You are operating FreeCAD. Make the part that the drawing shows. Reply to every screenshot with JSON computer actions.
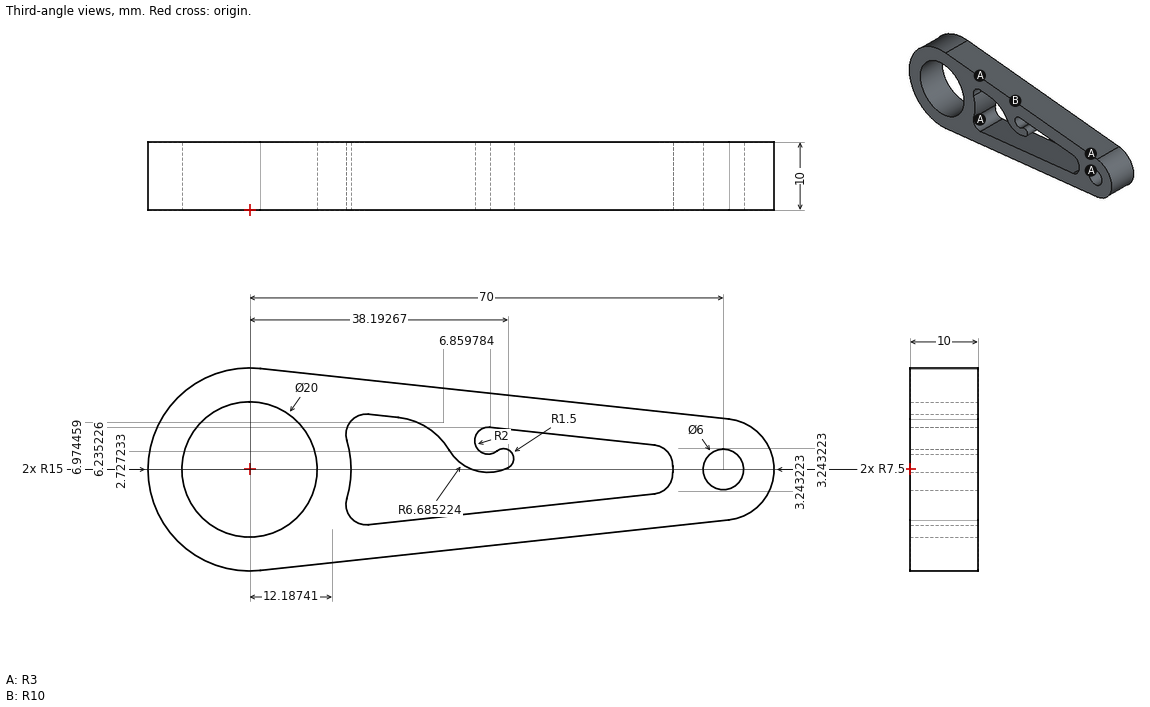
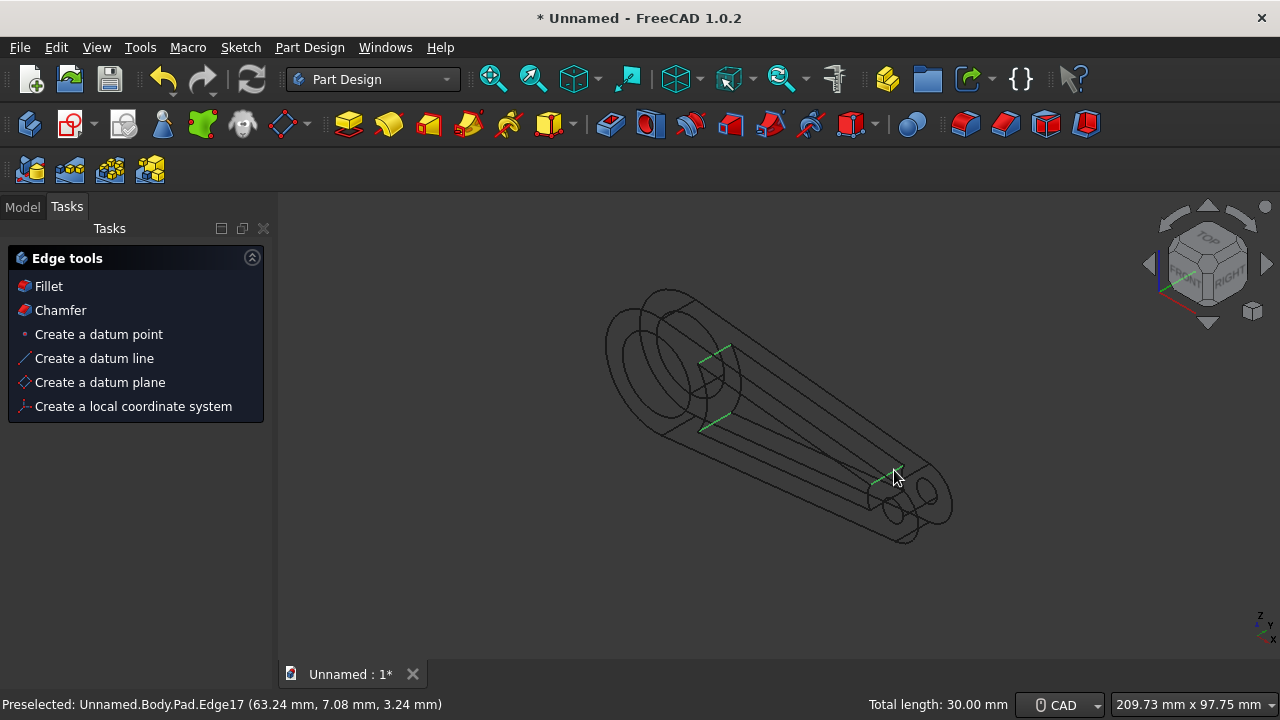
{"action": "scroll", "coordinate": [887, 500], "scroll_direction": "up", "scroll_amount": 6}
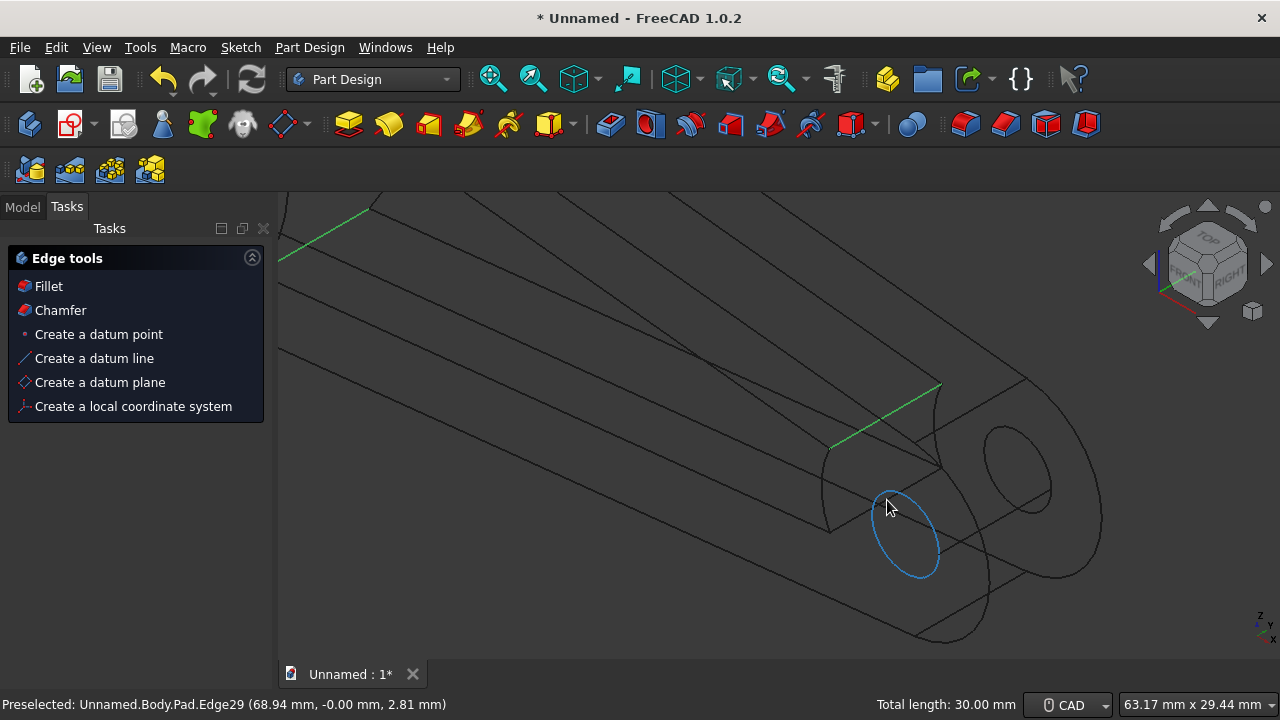
{"action": "left_click", "coordinate": [886, 499], "text": "ctrl"}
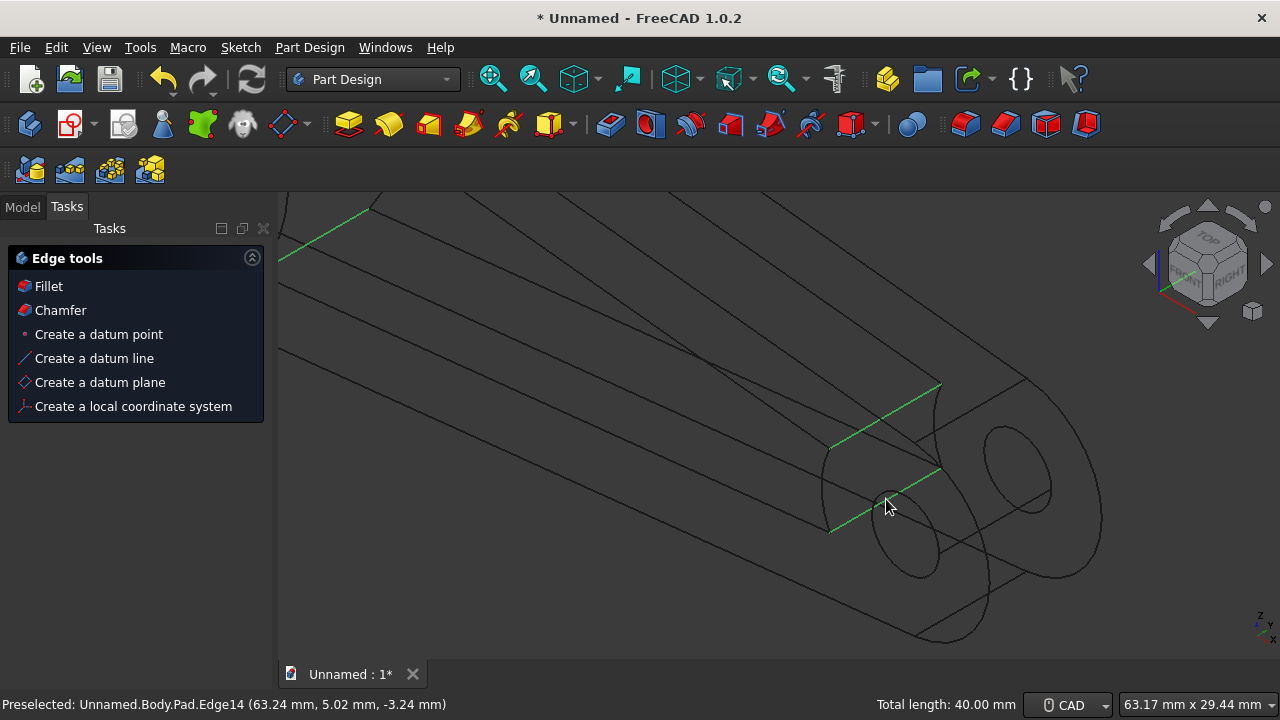
{"action": "key", "text": "v 1"}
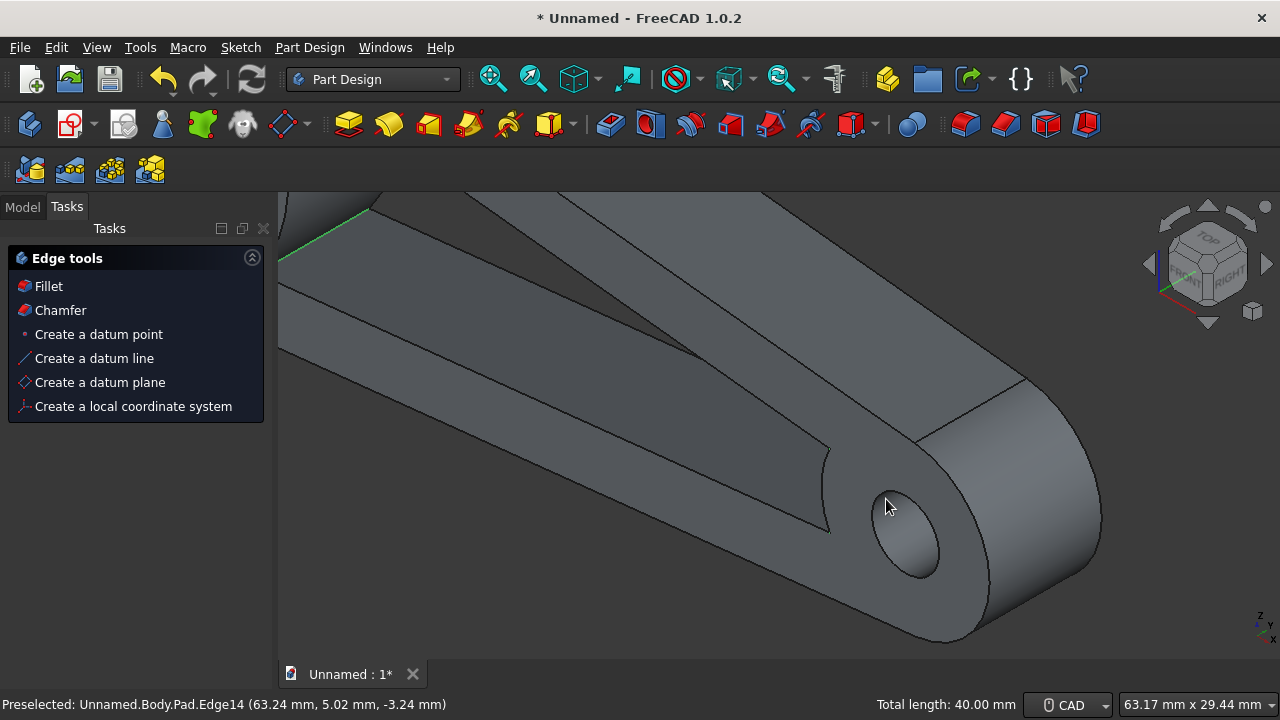
{"action": "left_click", "coordinate": [966, 124]}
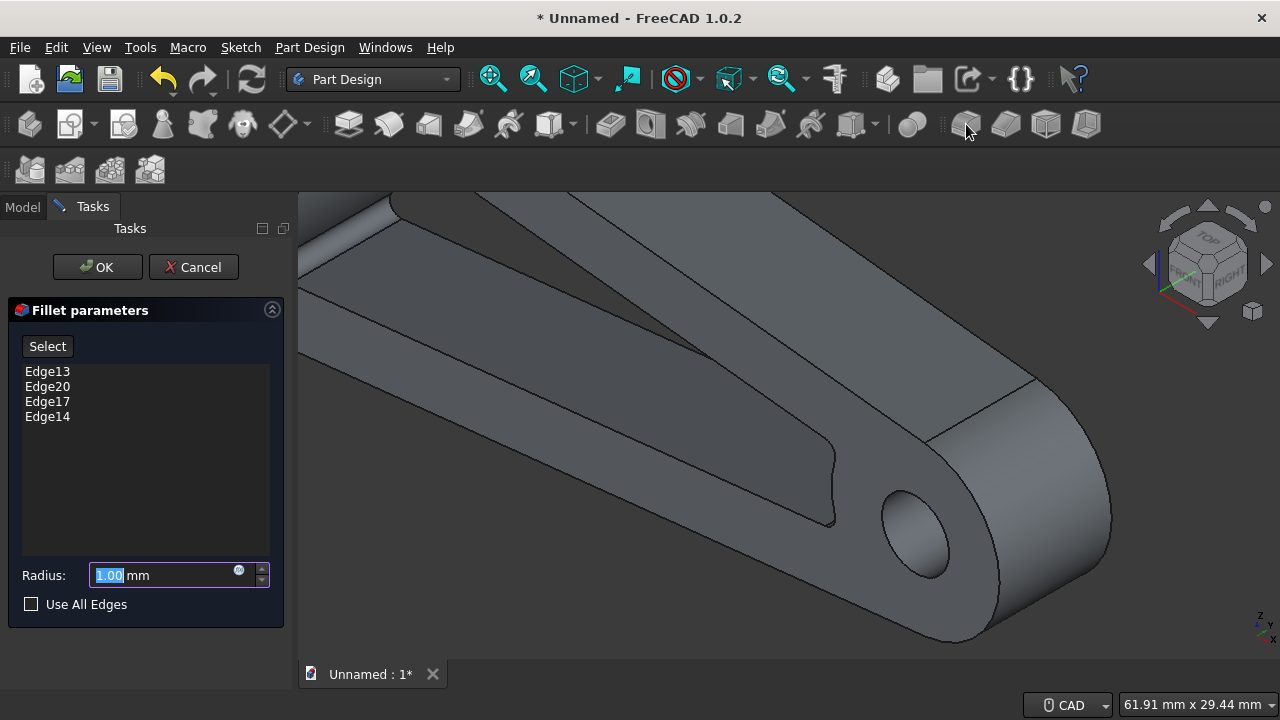
{"action": "type", "text": "3"}
{"action": "key", "text": "Tab"}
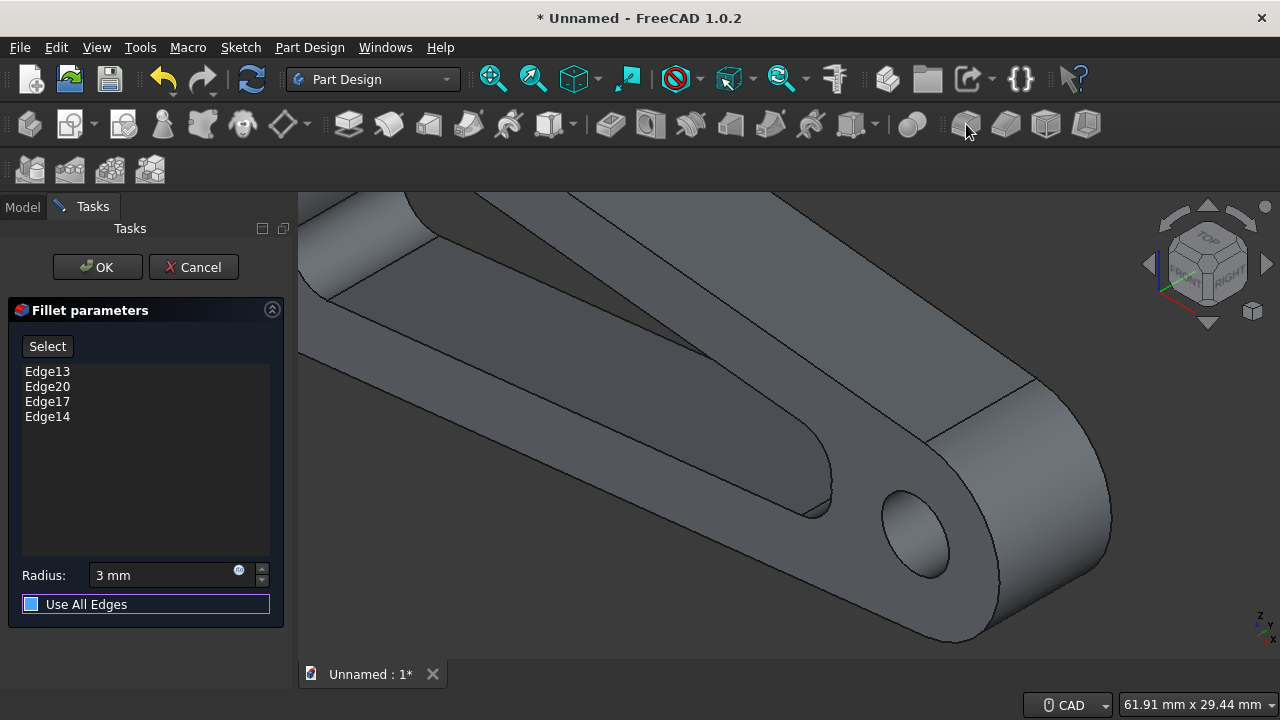
{"action": "left_click", "coordinate": [98, 267]}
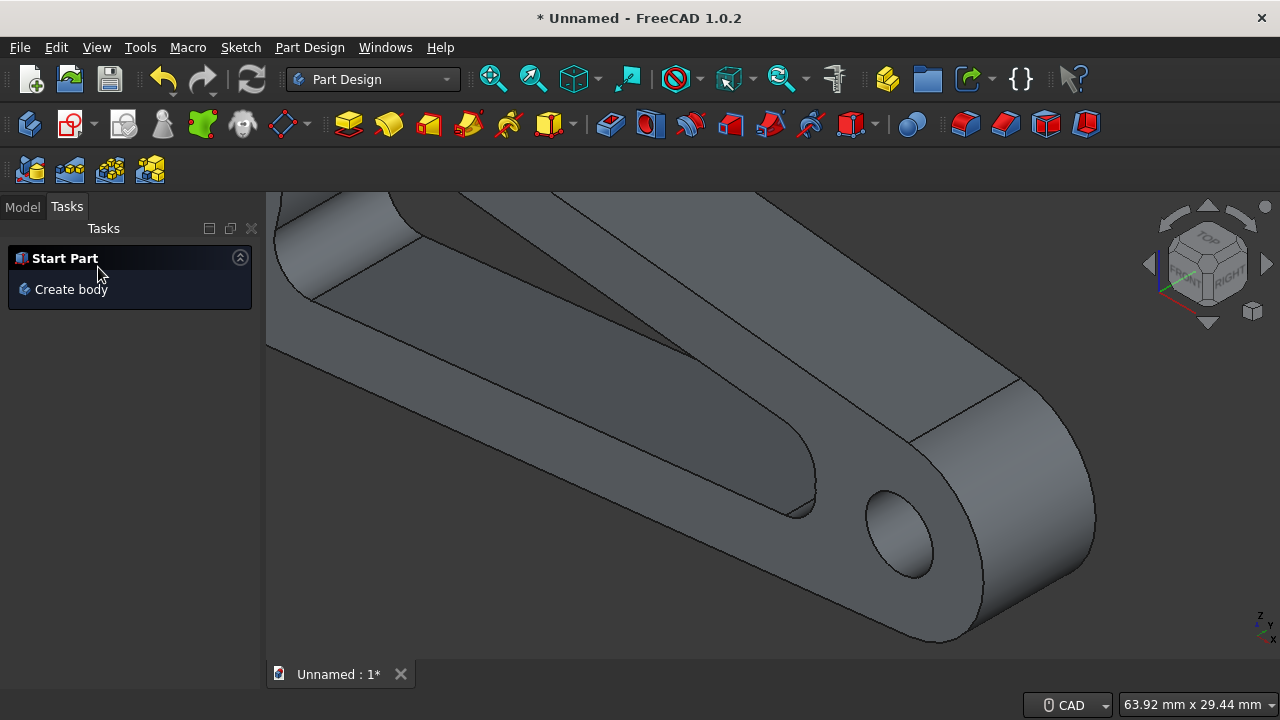
{"action": "left_click", "coordinate": [494, 80]}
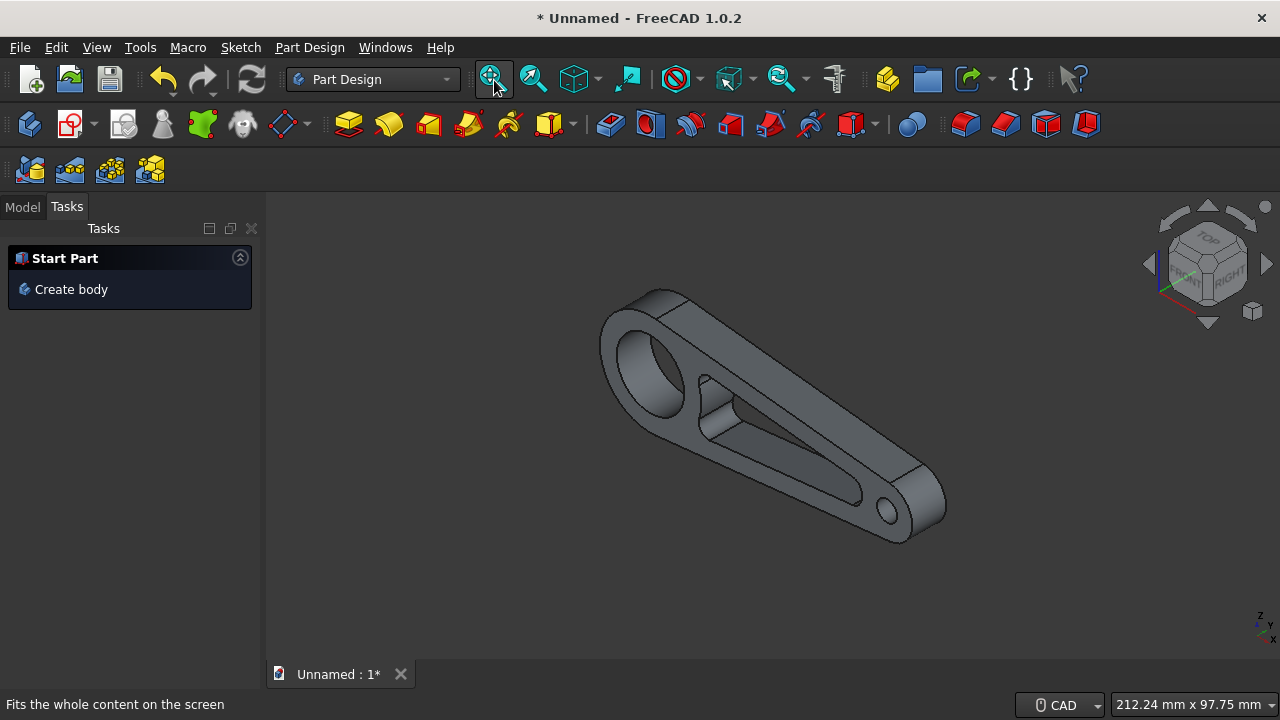
{"action": "key", "text": "4"}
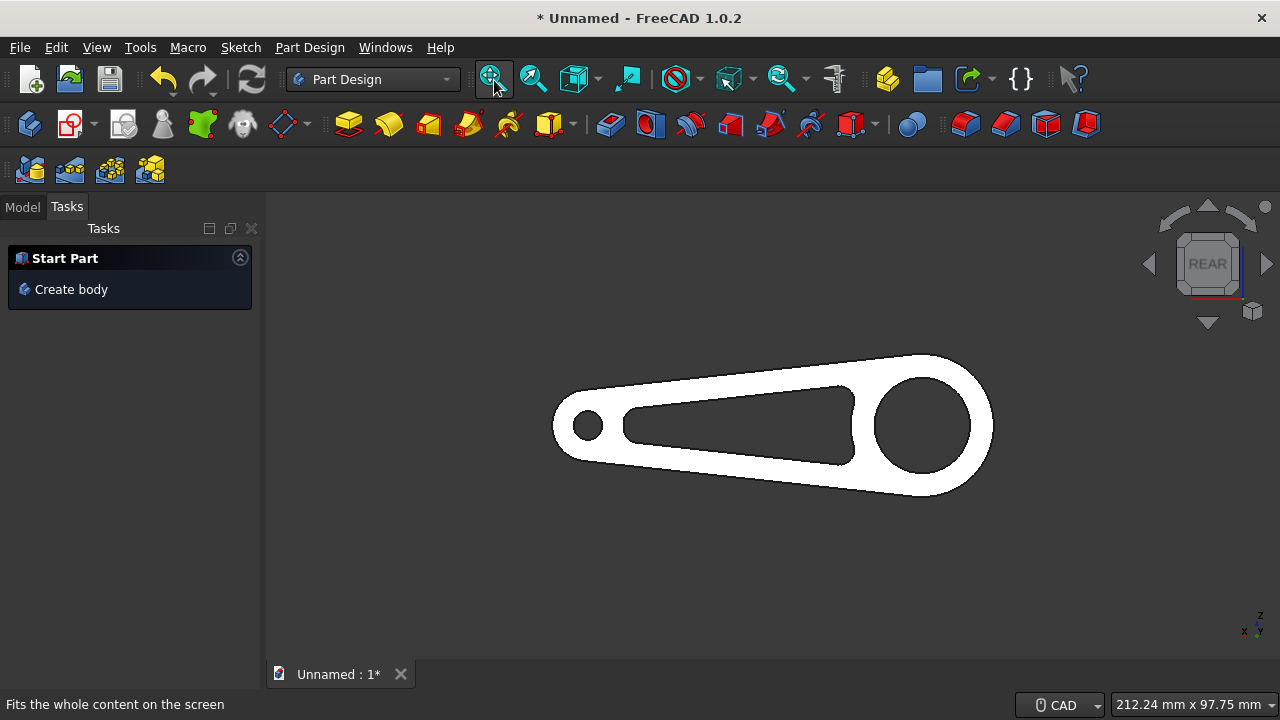
{"action": "left_click", "coordinate": [494, 80]}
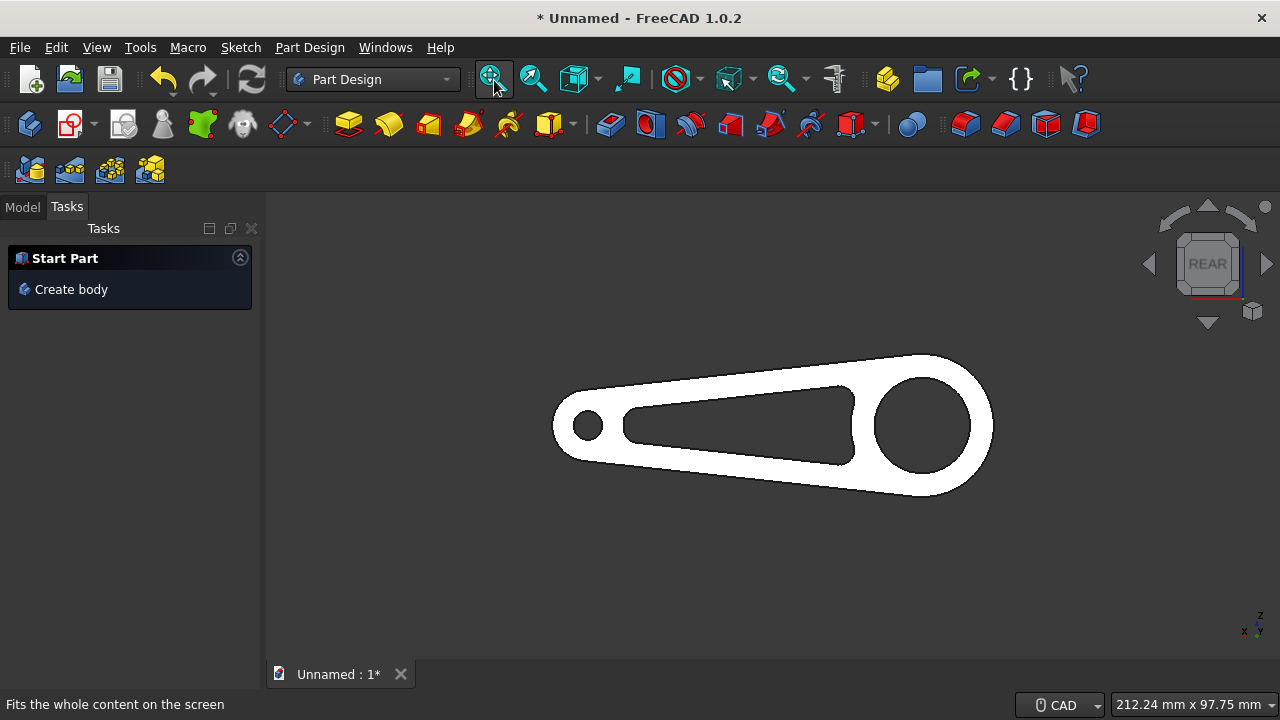
{"action": "left_click", "coordinate": [962, 465]}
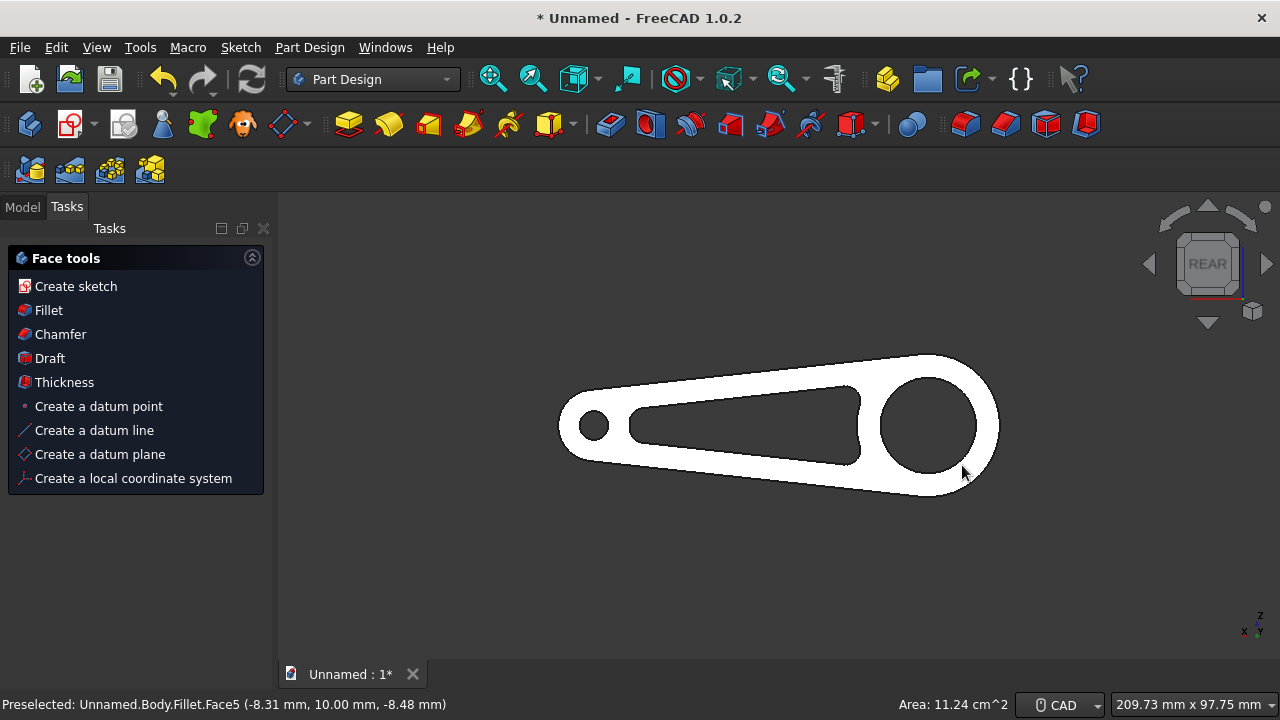
{"action": "left_click", "coordinate": [70, 124]}